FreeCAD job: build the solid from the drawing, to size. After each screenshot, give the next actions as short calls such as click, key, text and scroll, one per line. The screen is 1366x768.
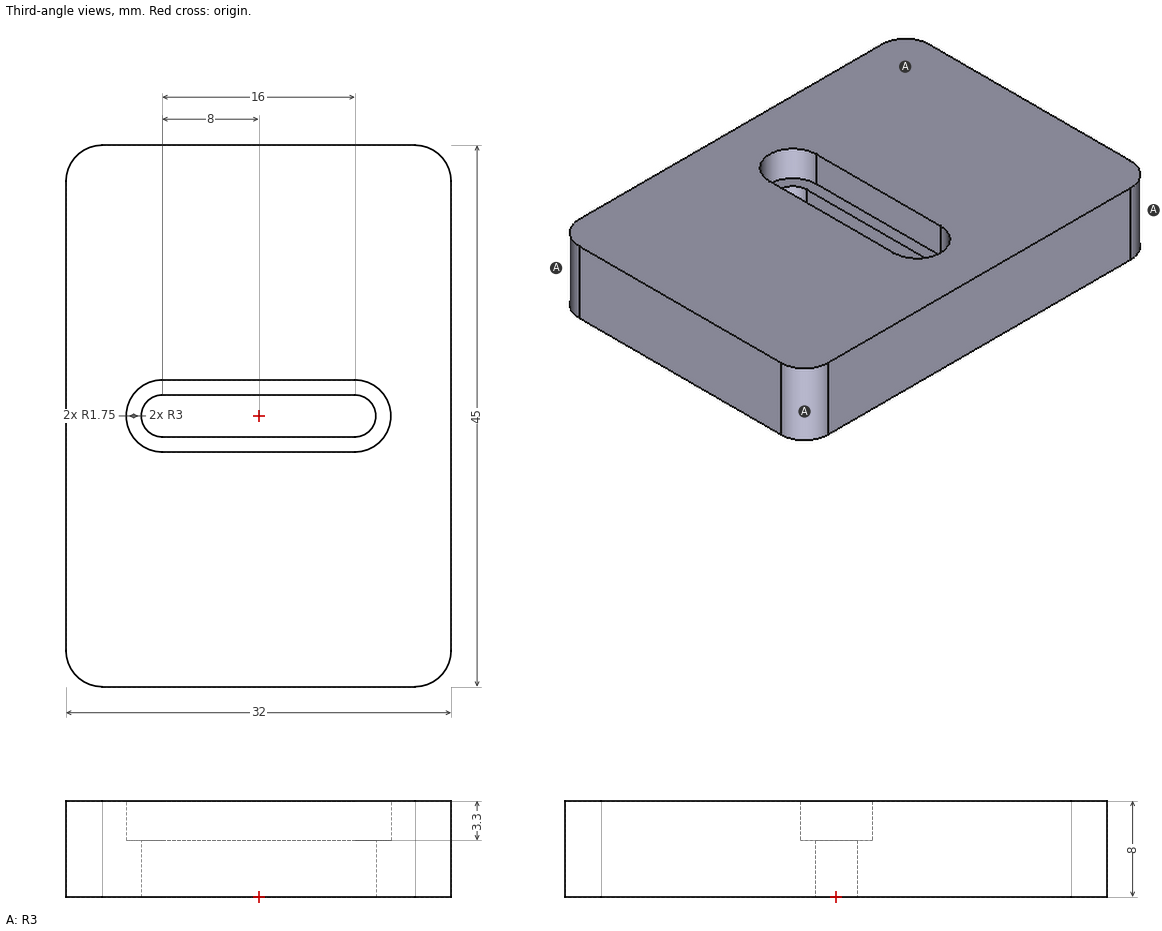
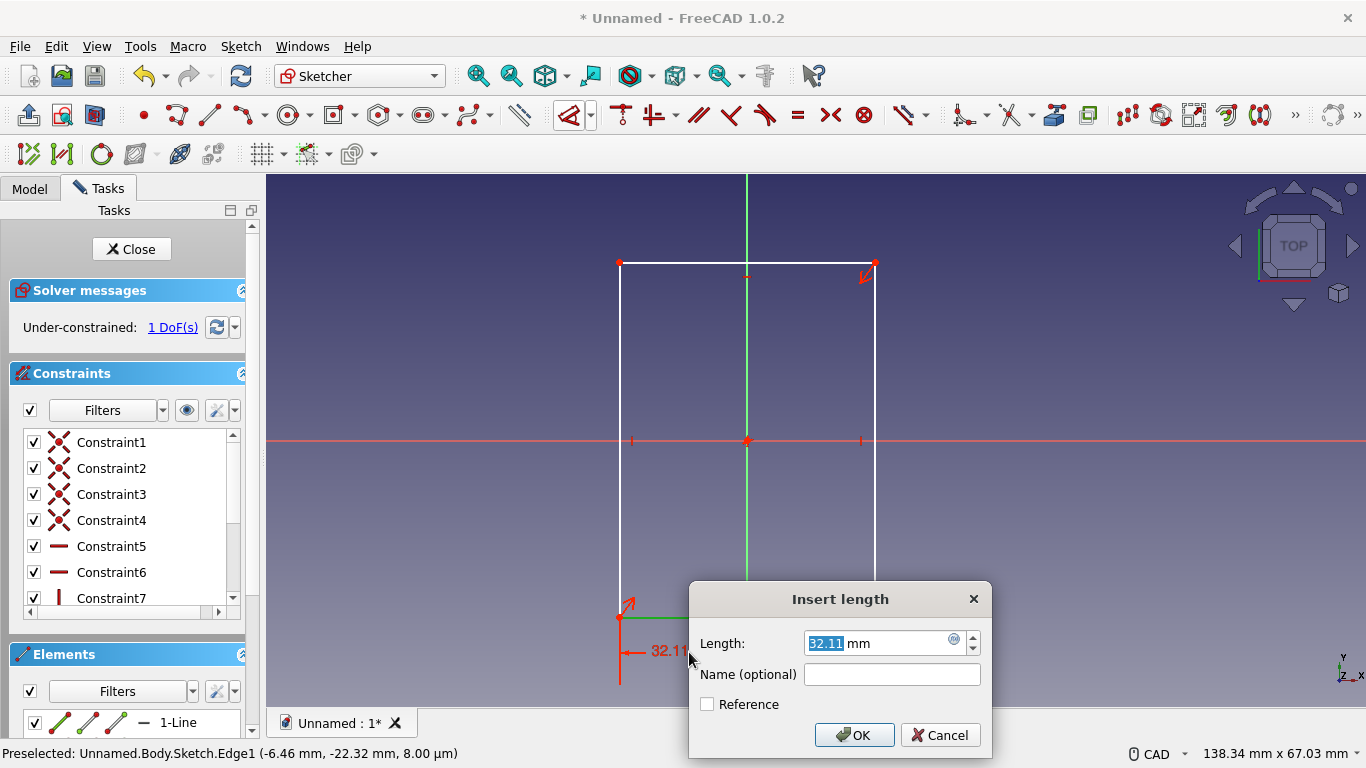
text(32)
key(Return)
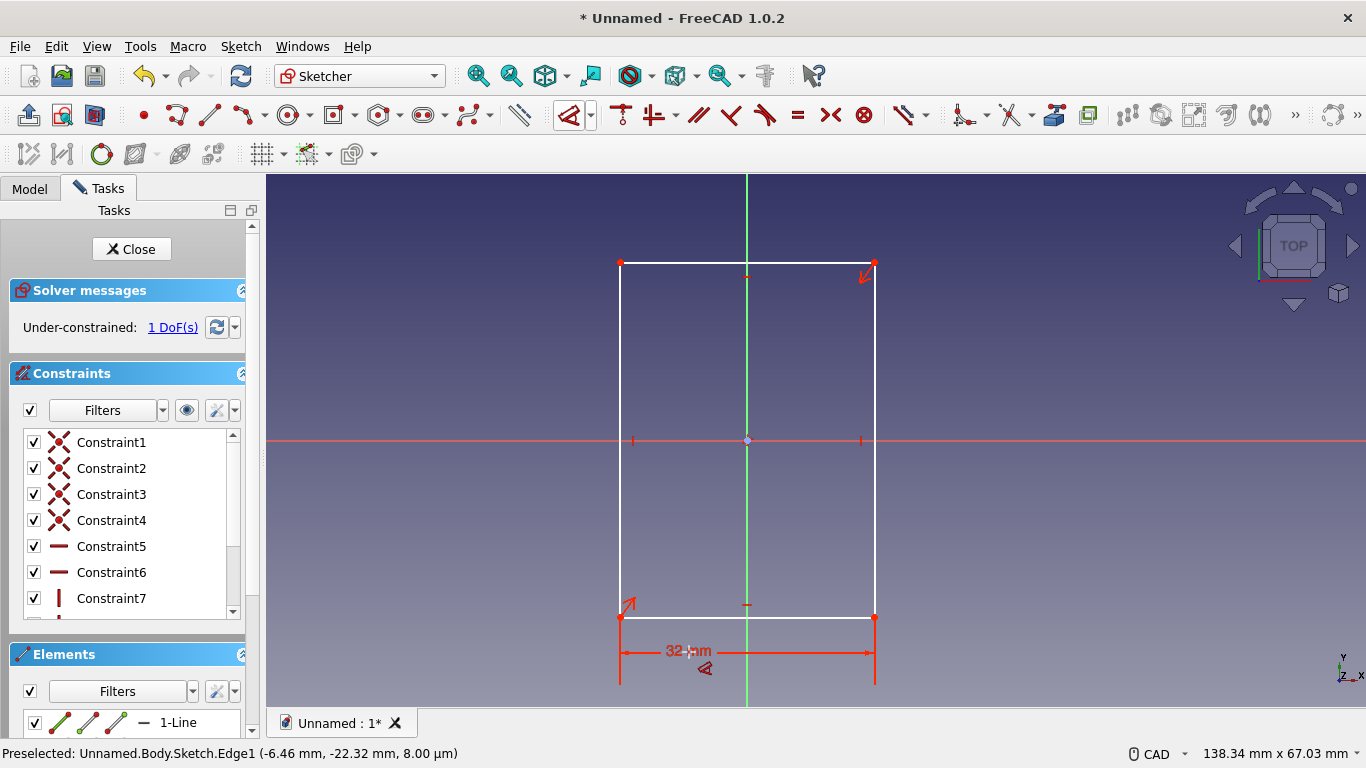
click(875, 511)
click(909, 359)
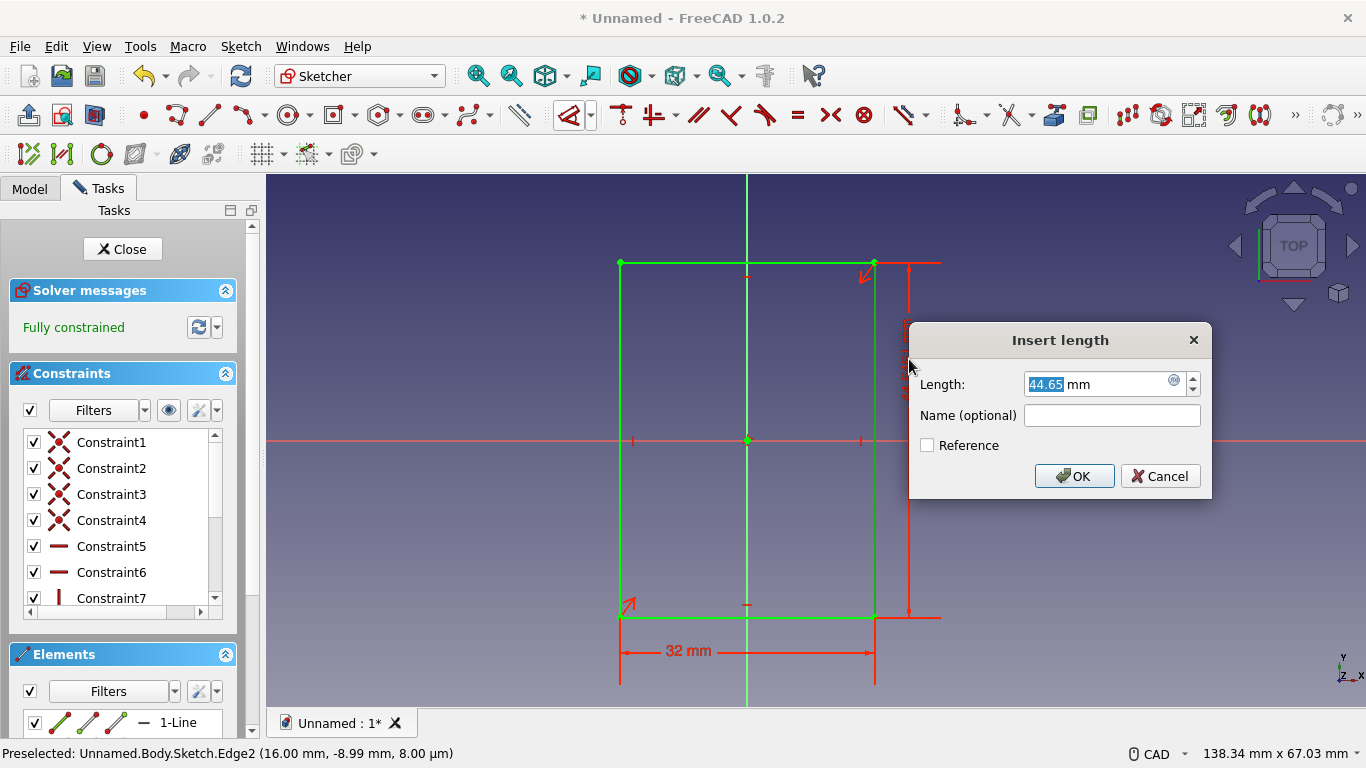
text(45)
key(Return)
key(Escape)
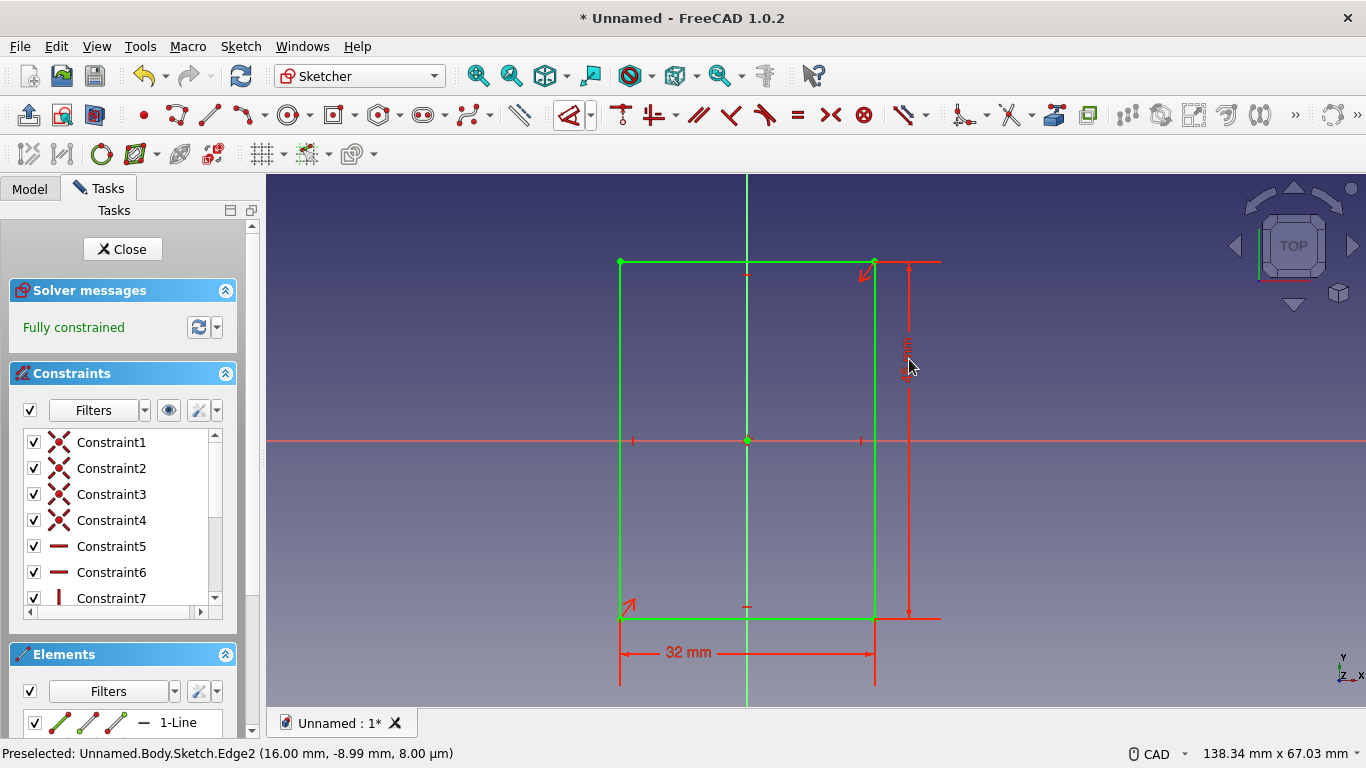
click(123, 249)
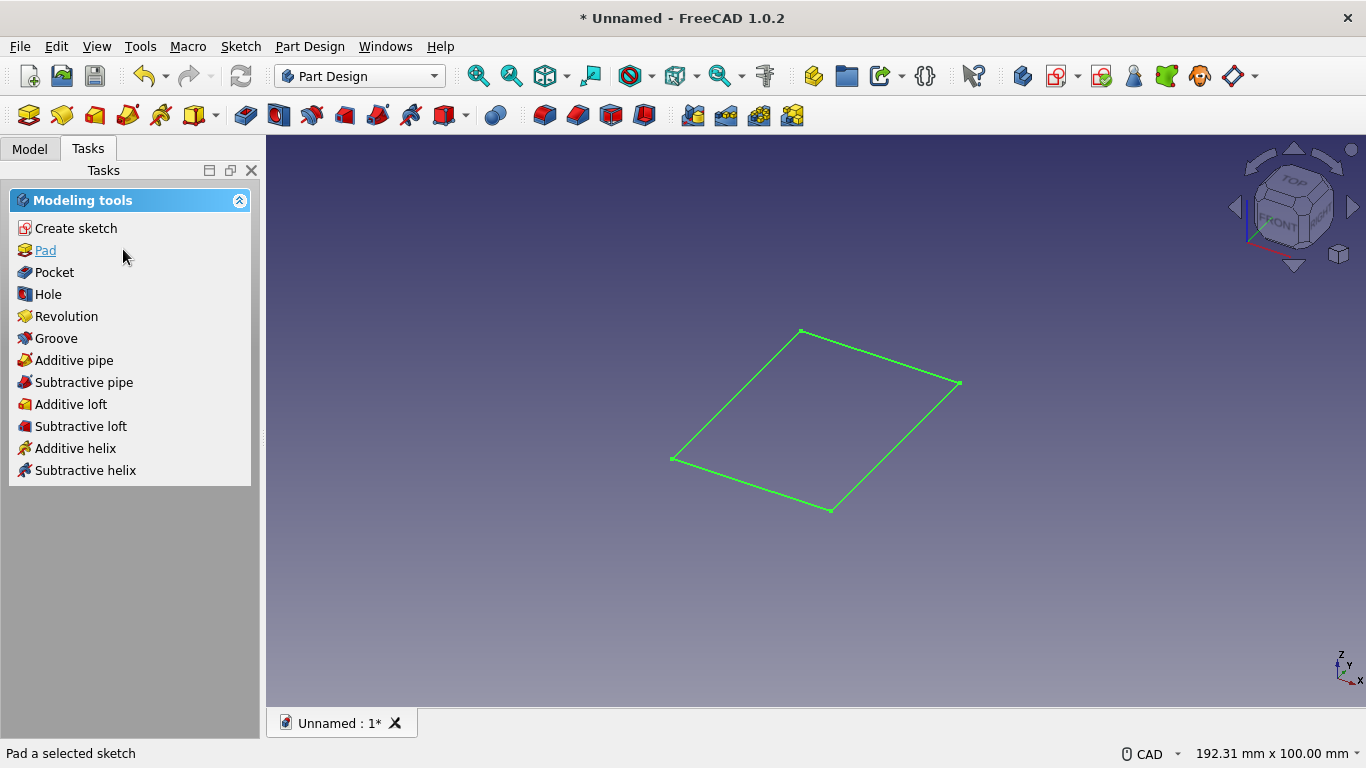
click(29, 116)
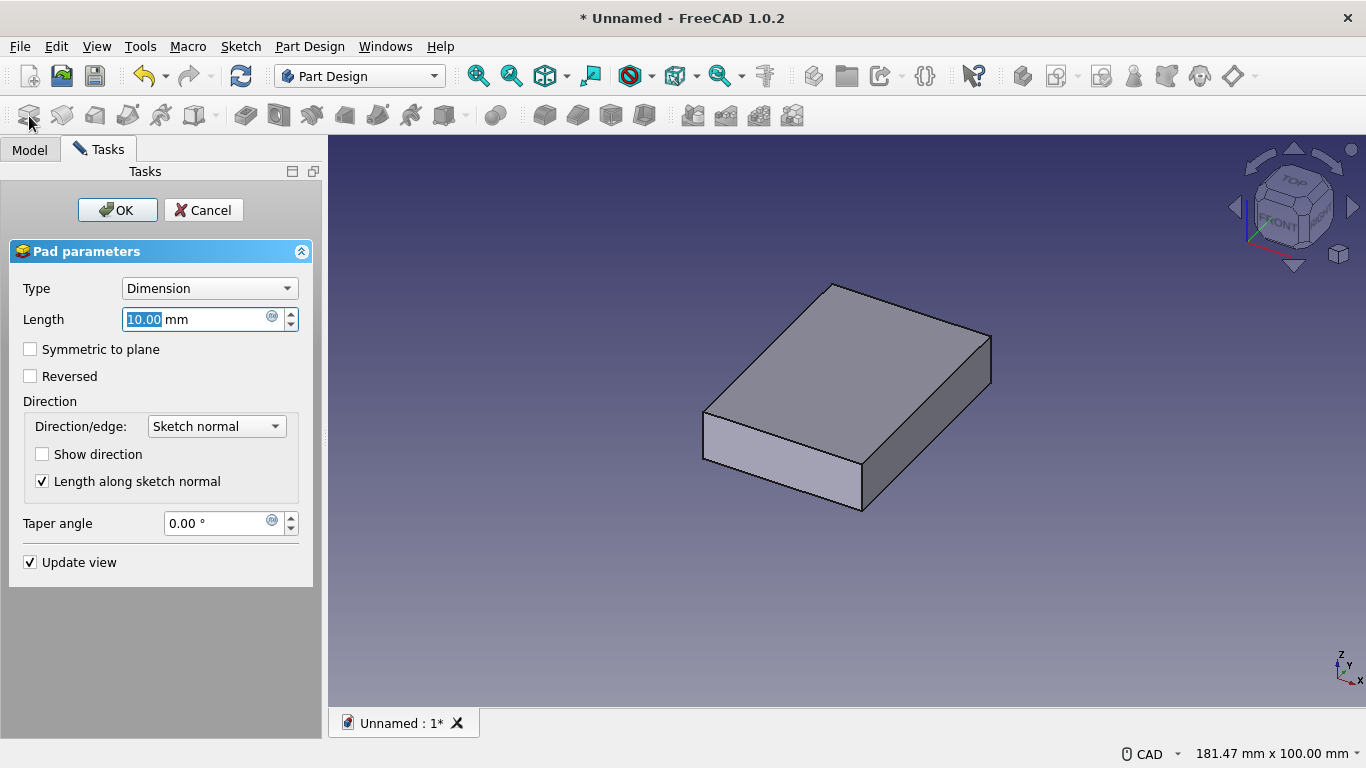
text(8)
key(Tab)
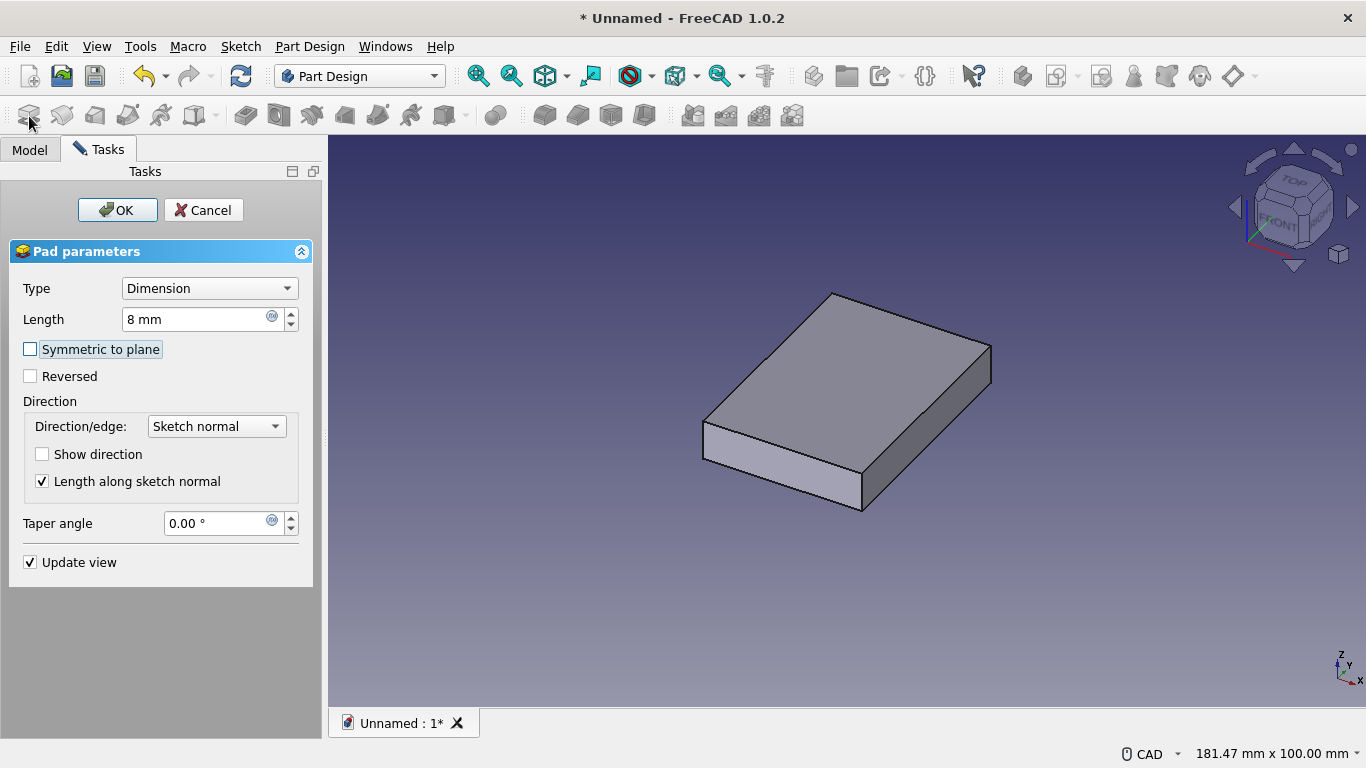
click(118, 210)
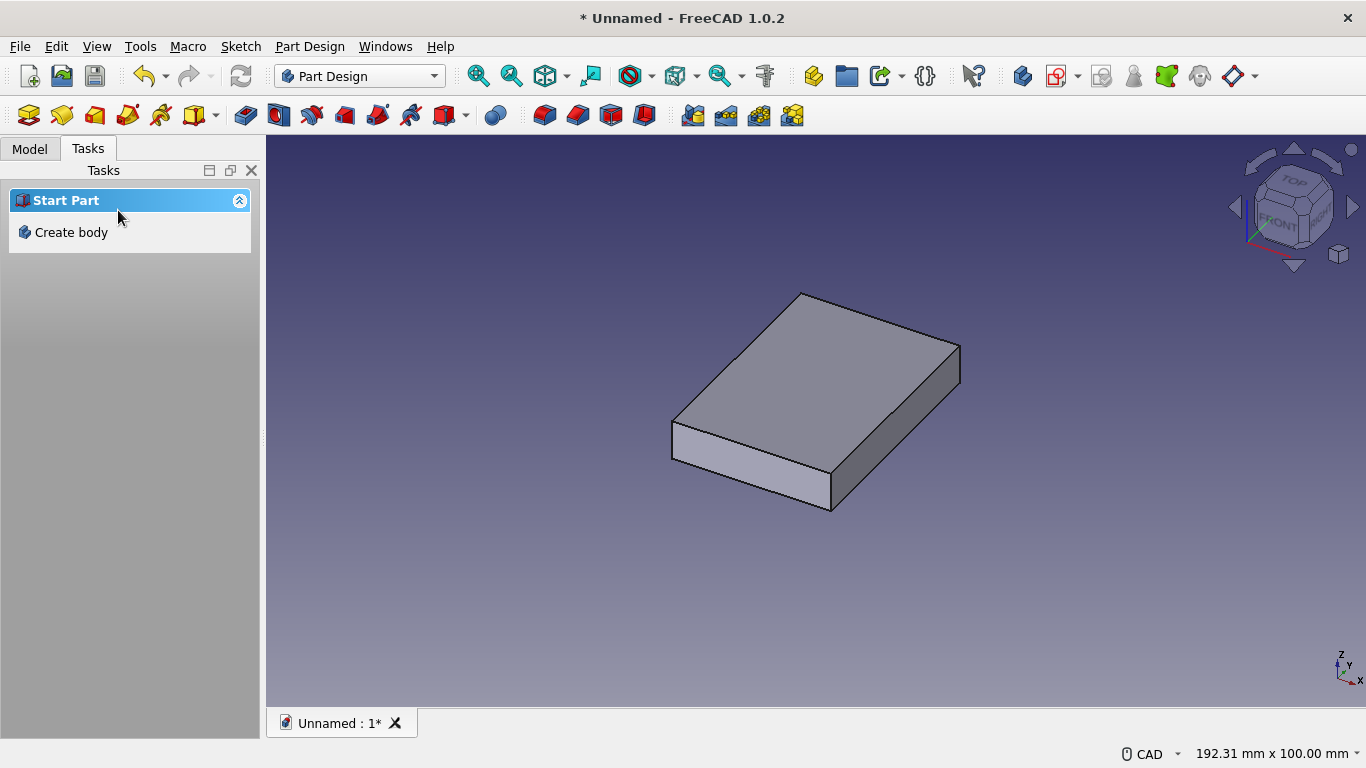
key(v)
key(f)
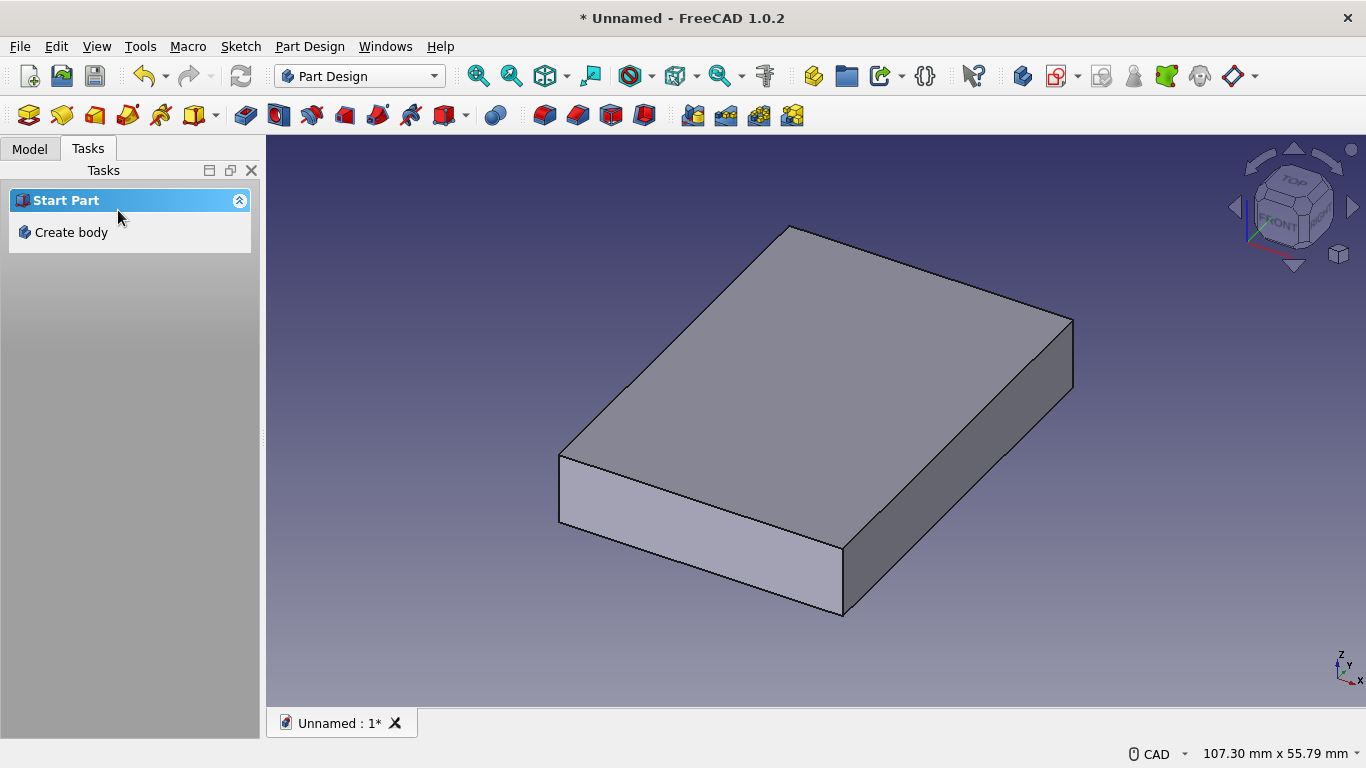
click(849, 354)